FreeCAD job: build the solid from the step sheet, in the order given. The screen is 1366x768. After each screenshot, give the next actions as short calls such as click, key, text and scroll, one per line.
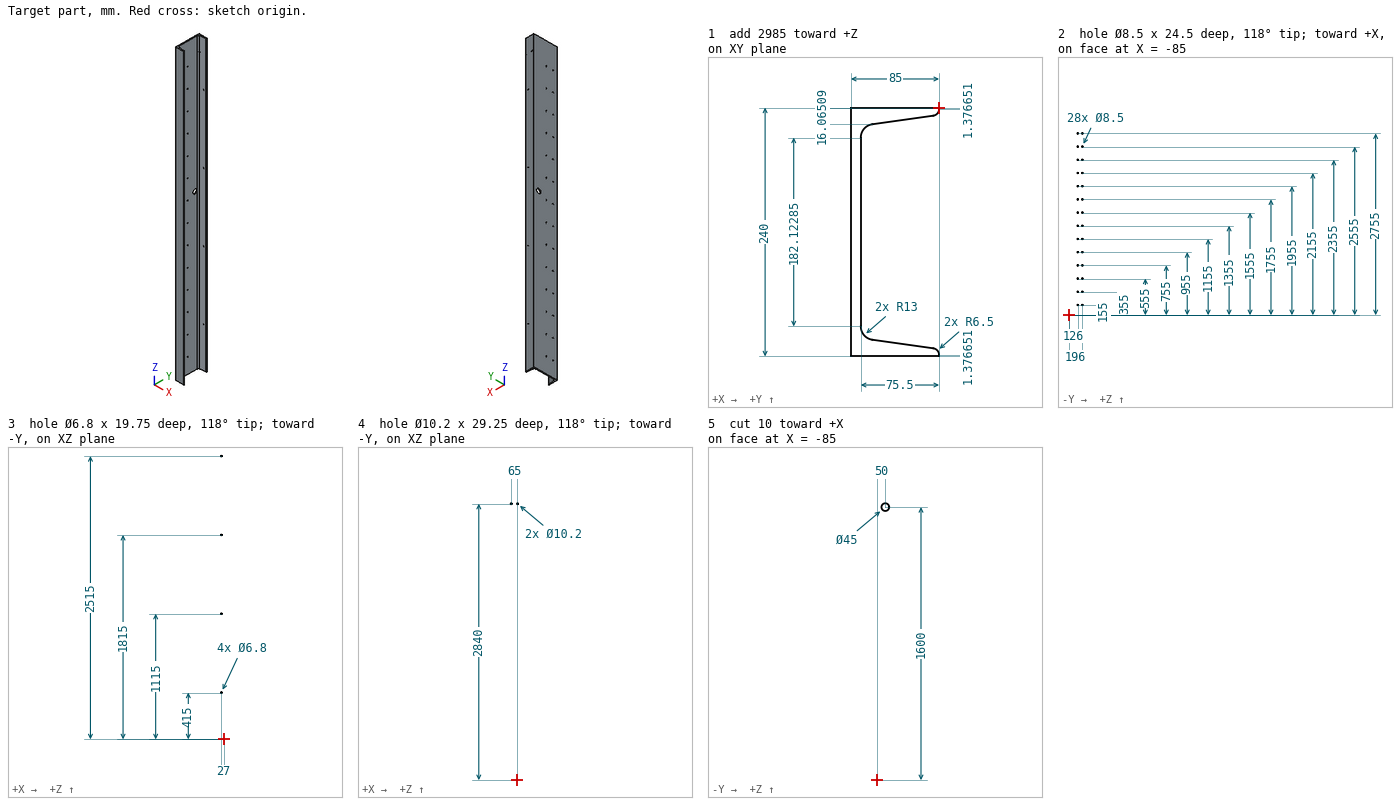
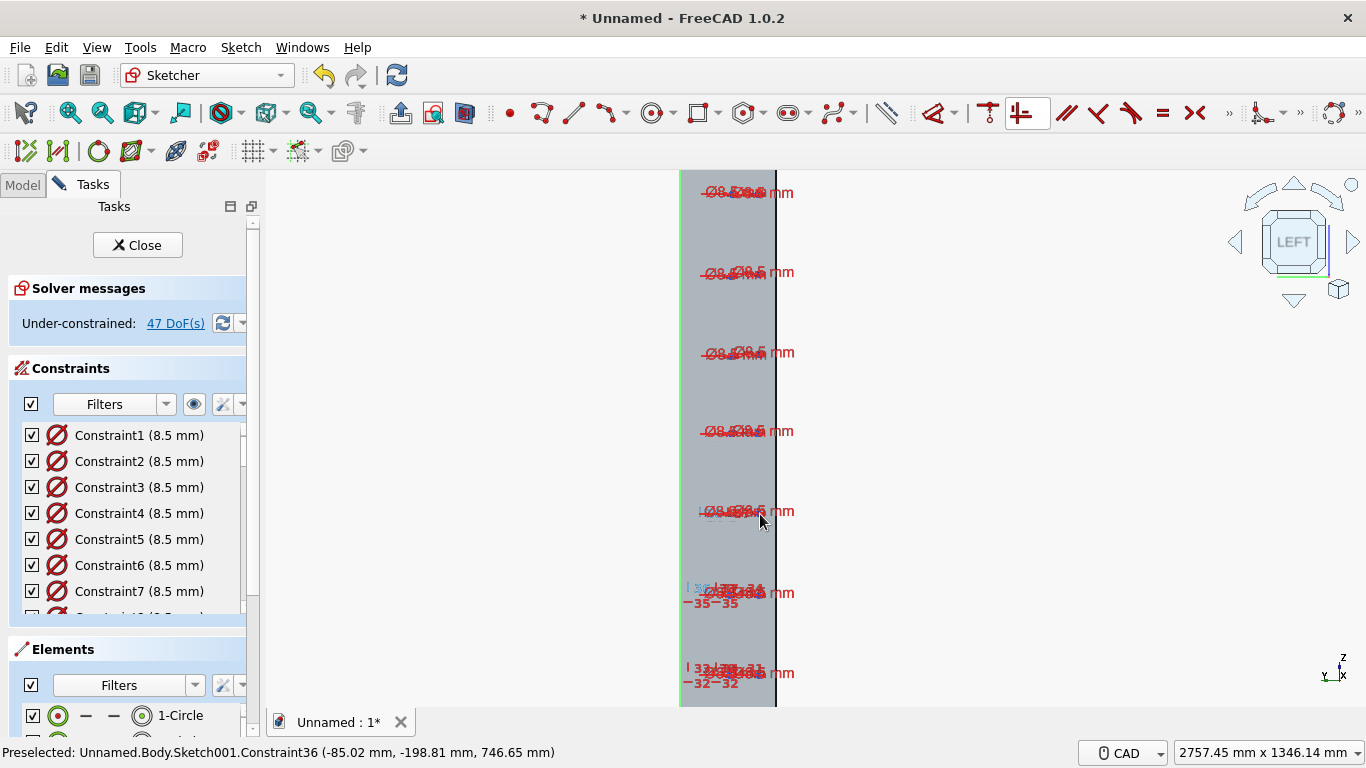
click(758, 513)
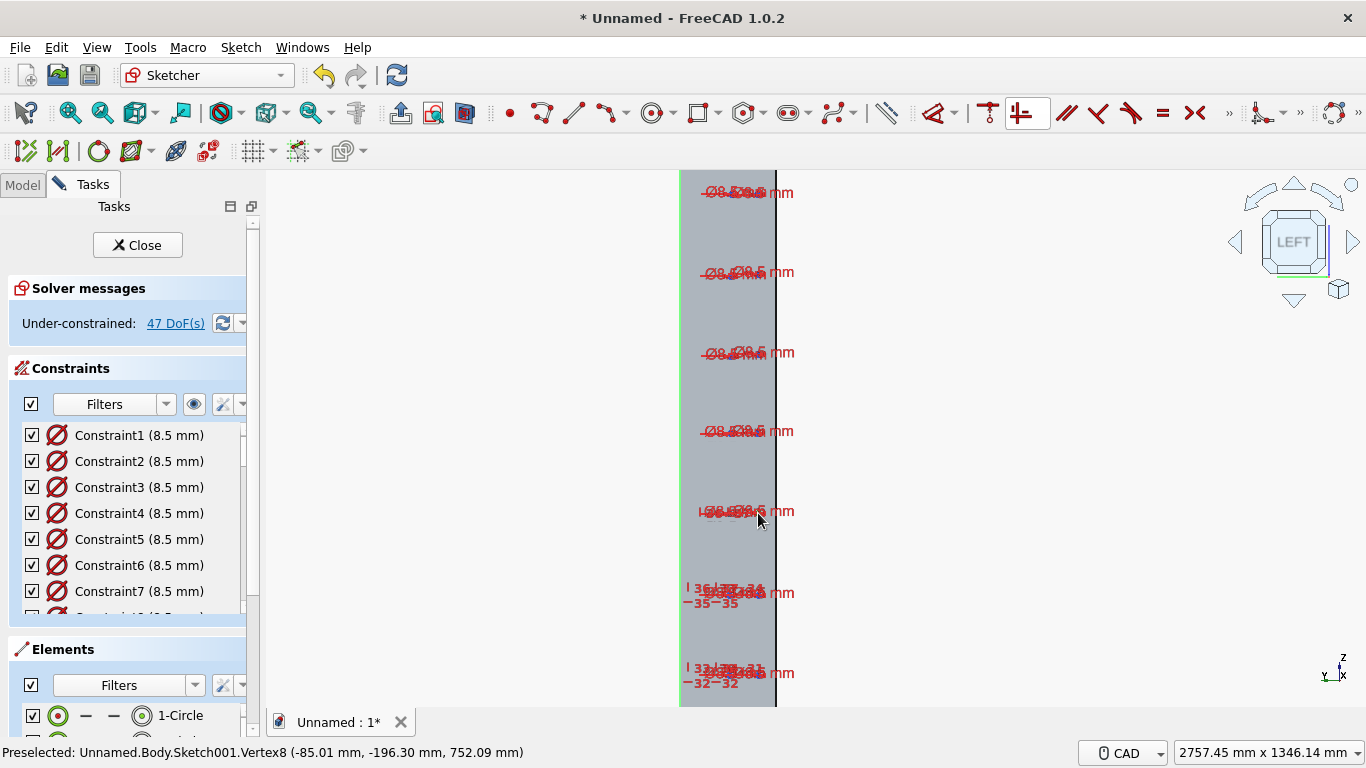
click(1044, 114)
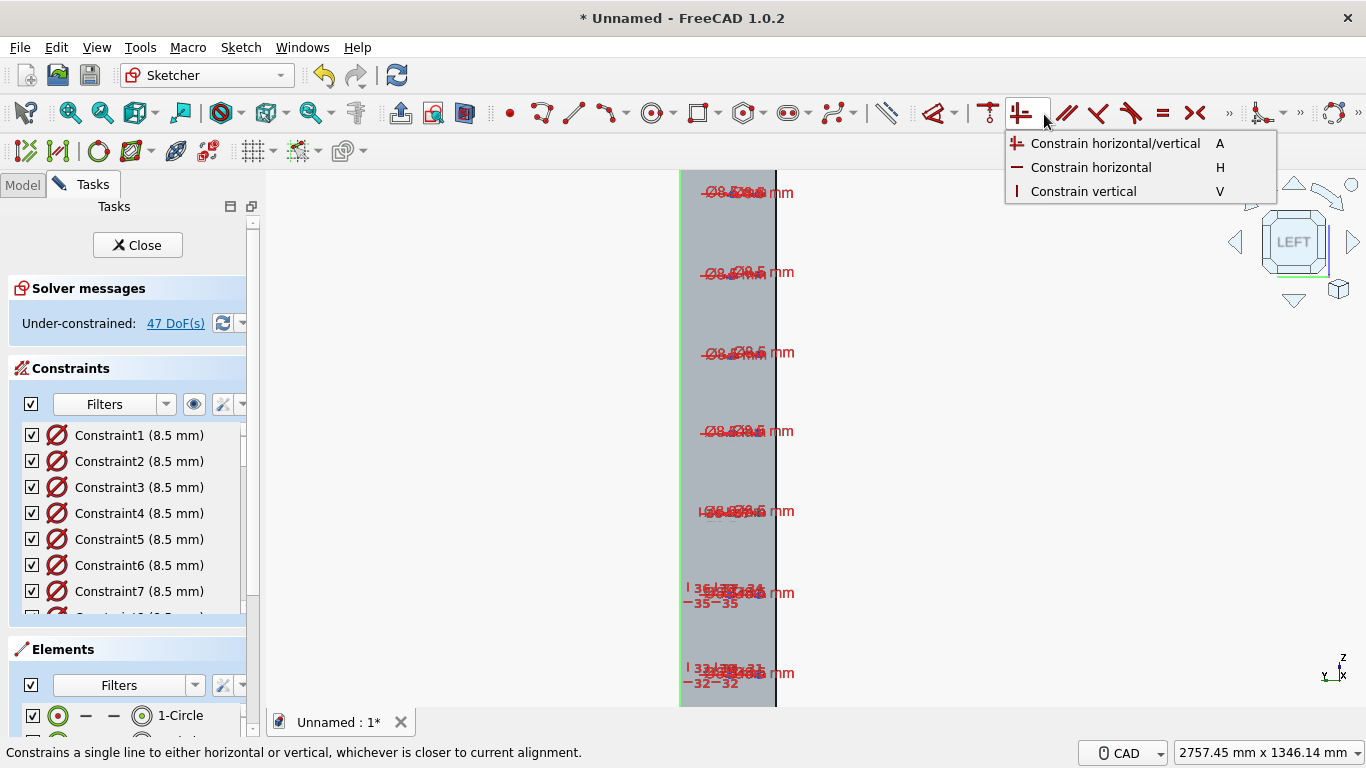
click(1141, 167)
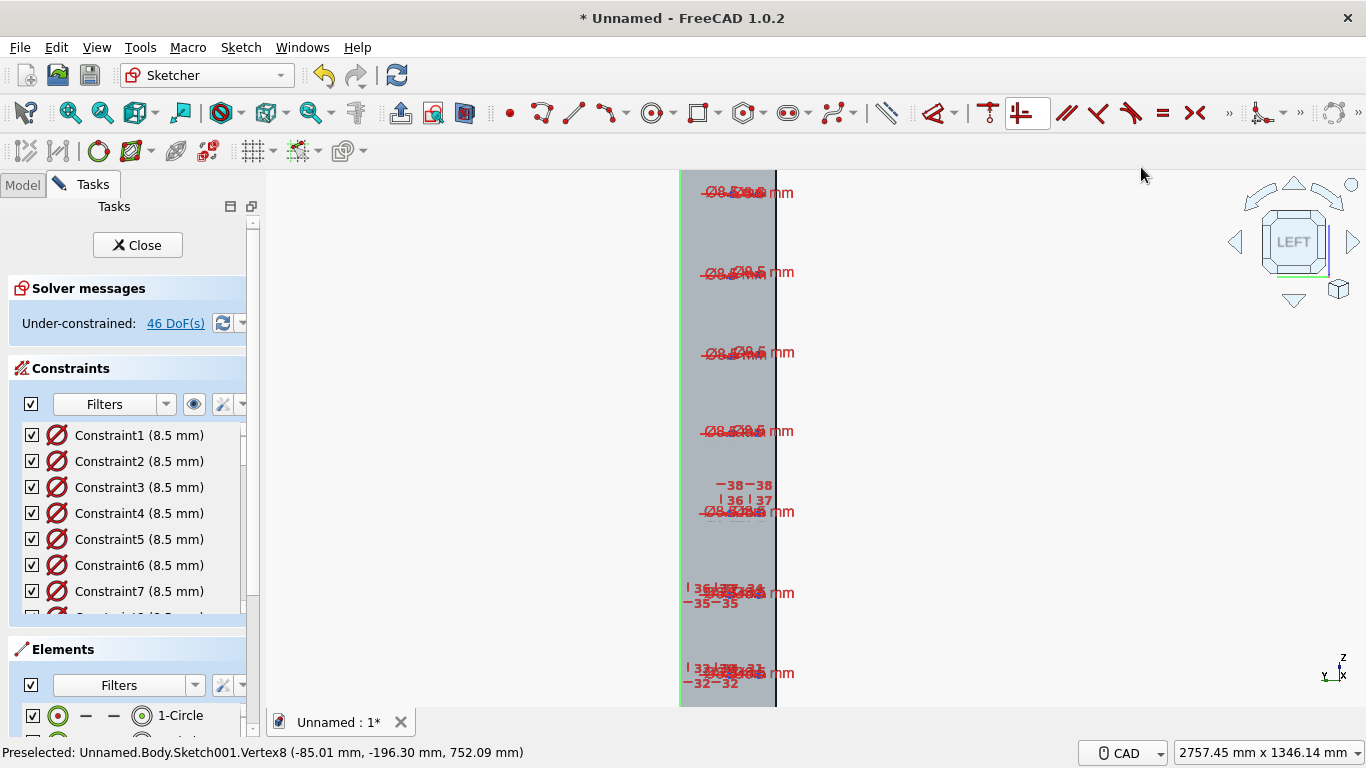
click(729, 514)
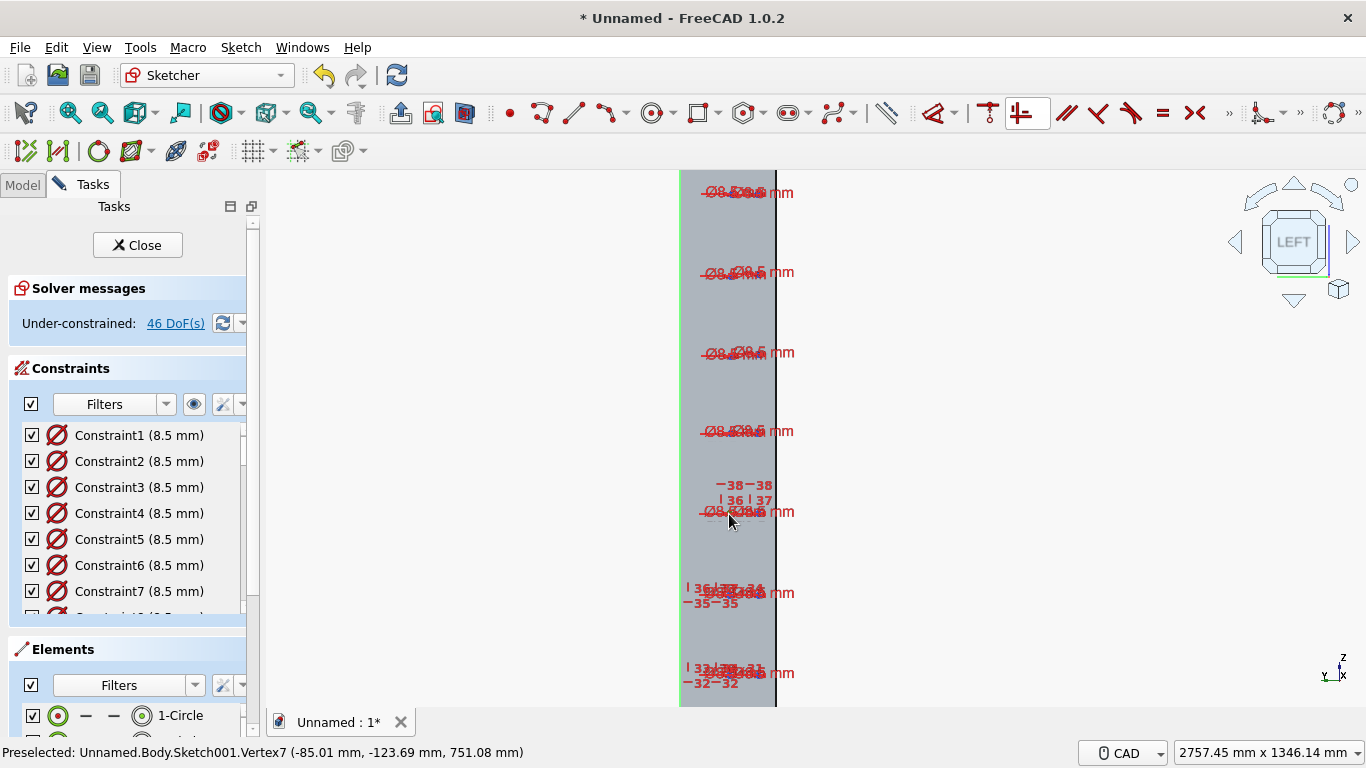
click(730, 434)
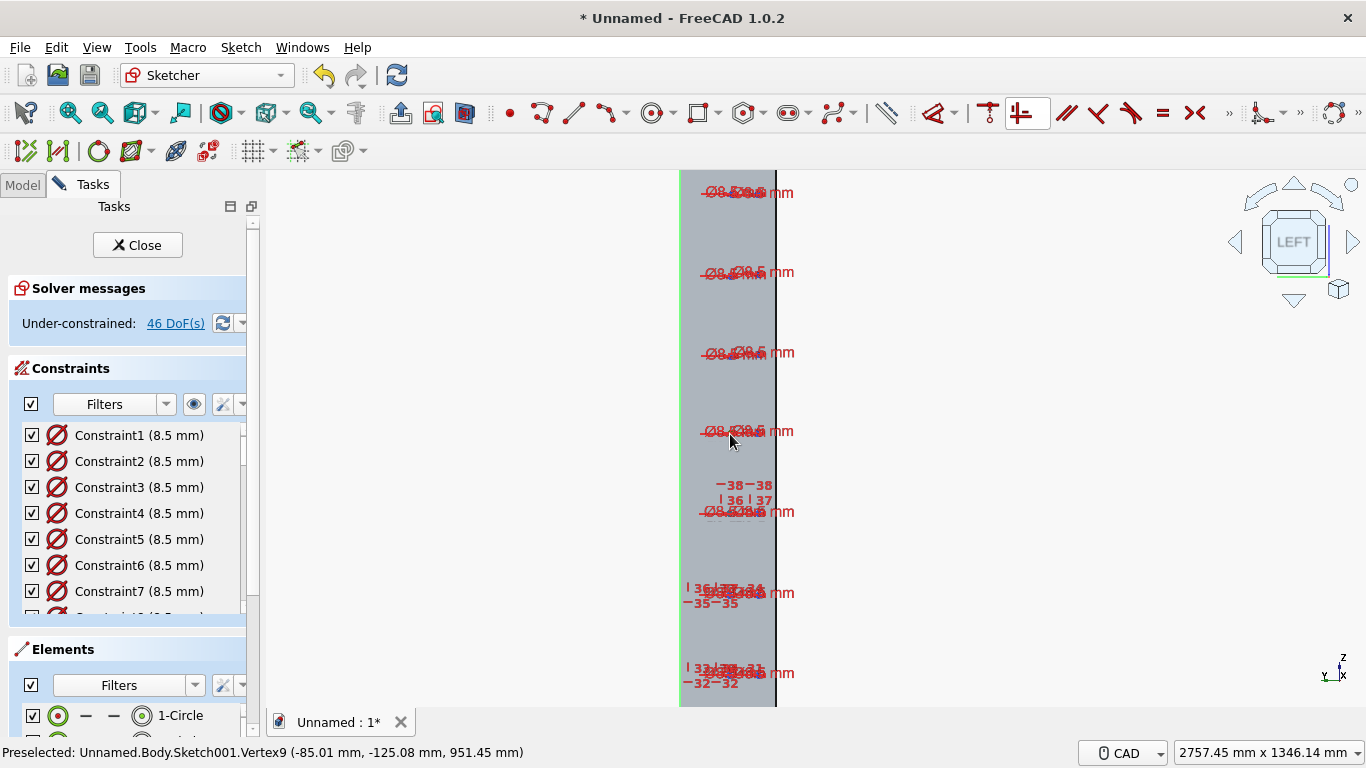
key(v)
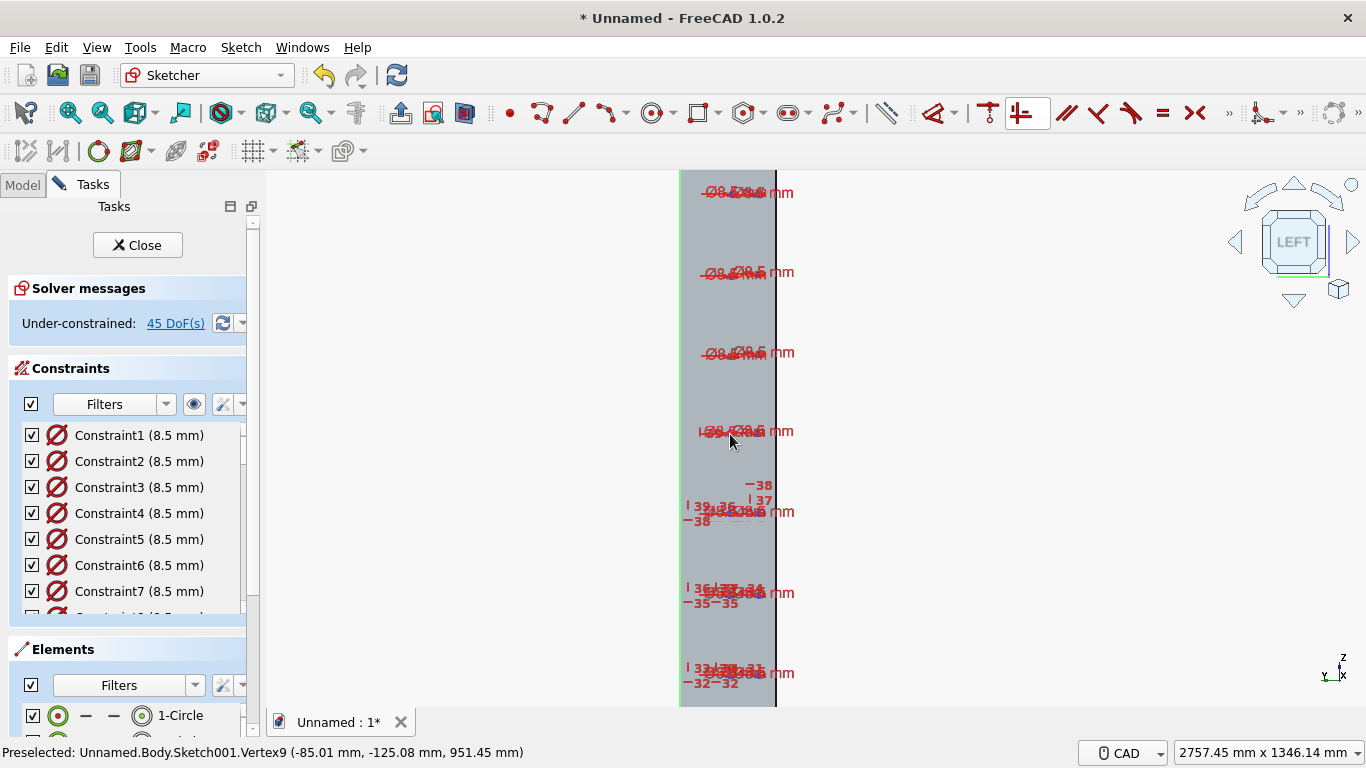
click(758, 514)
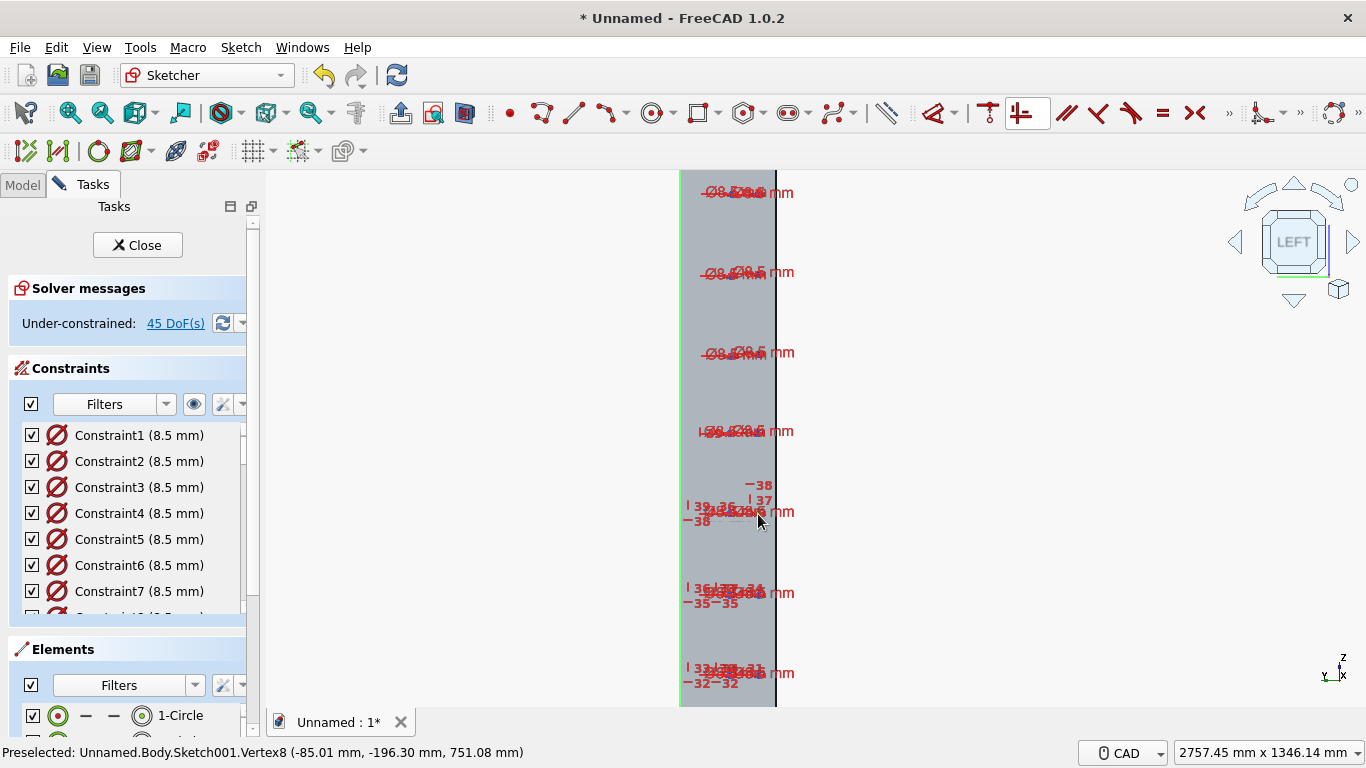
click(758, 433)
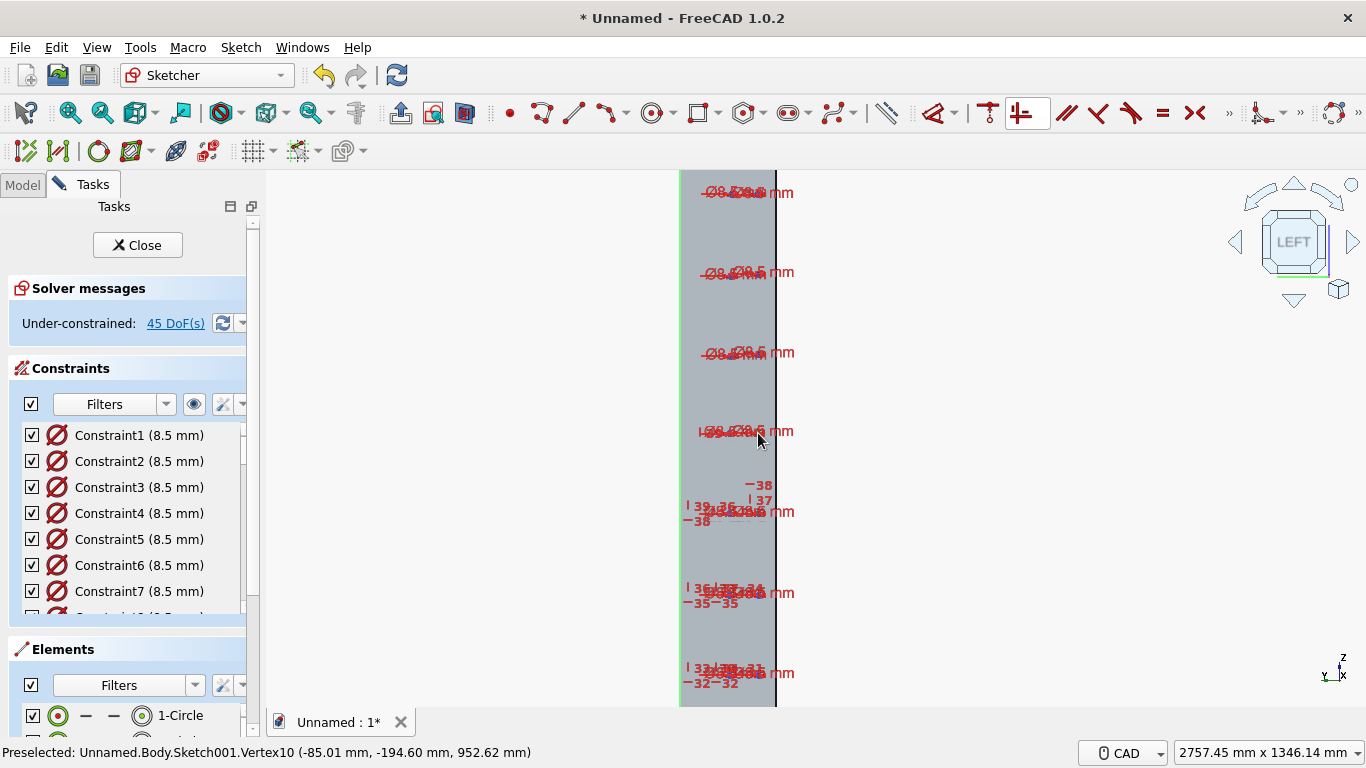
click(1044, 114)